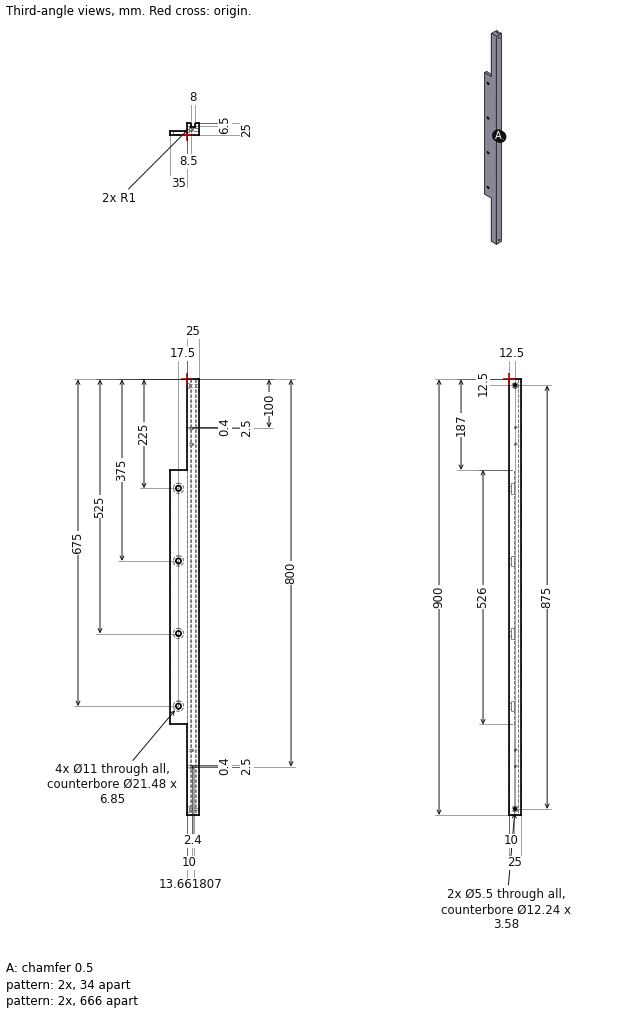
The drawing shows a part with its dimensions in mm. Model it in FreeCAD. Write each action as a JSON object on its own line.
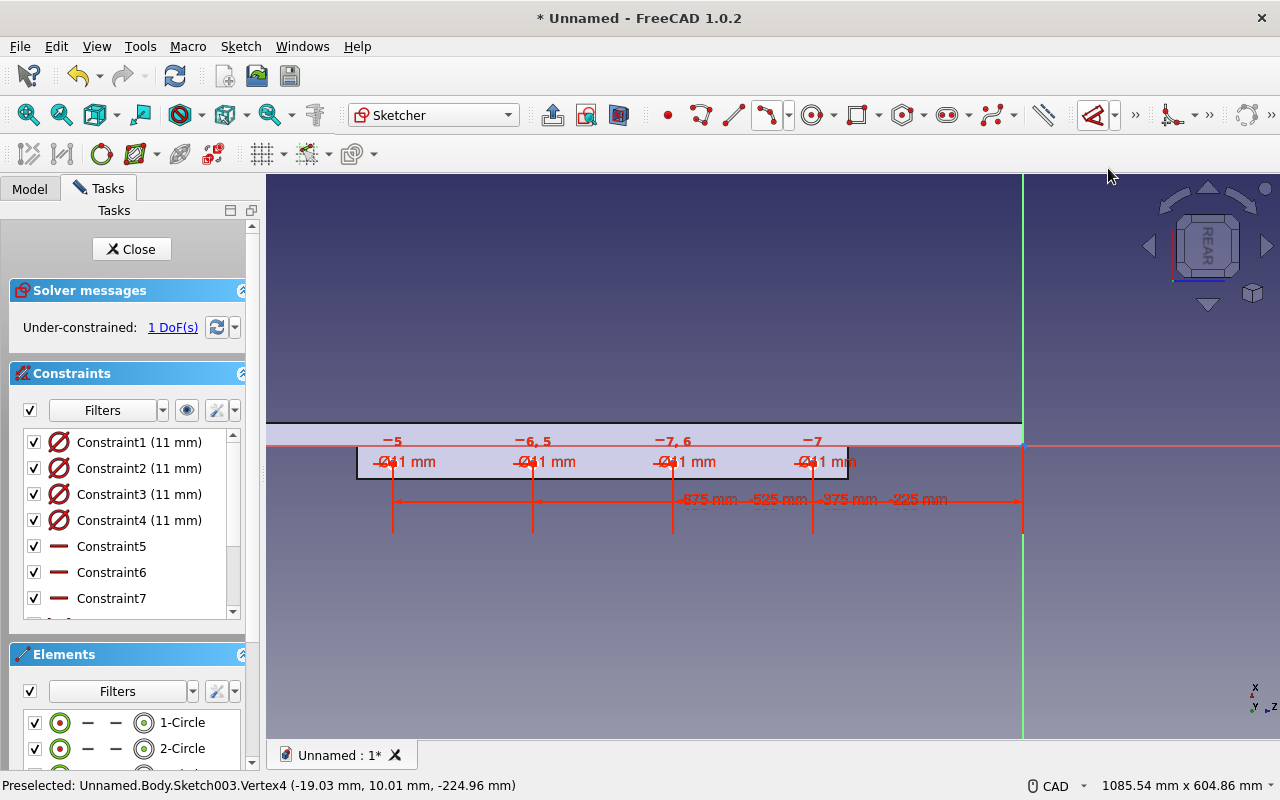
{"action": "scroll", "coordinate": [393, 464], "scroll_direction": "up", "scroll_amount": 5}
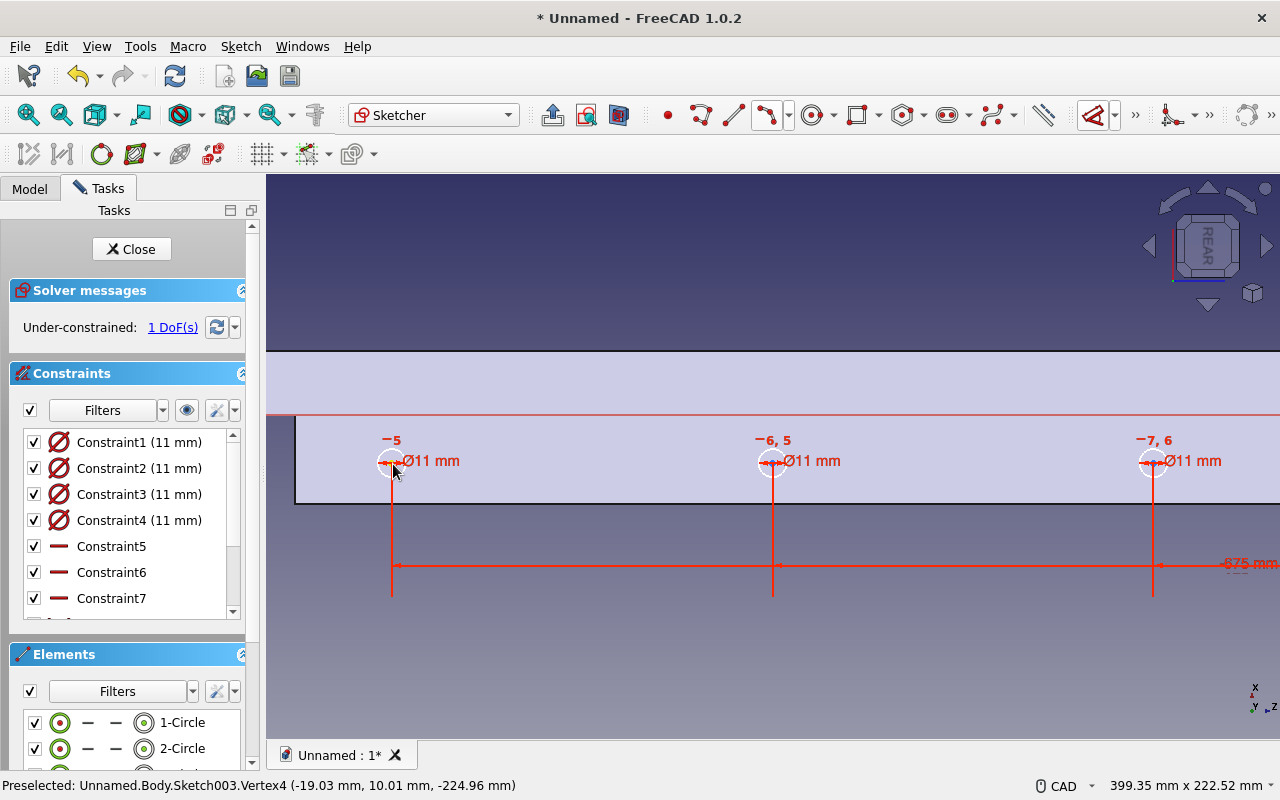
{"action": "left_click", "coordinate": [392, 463]}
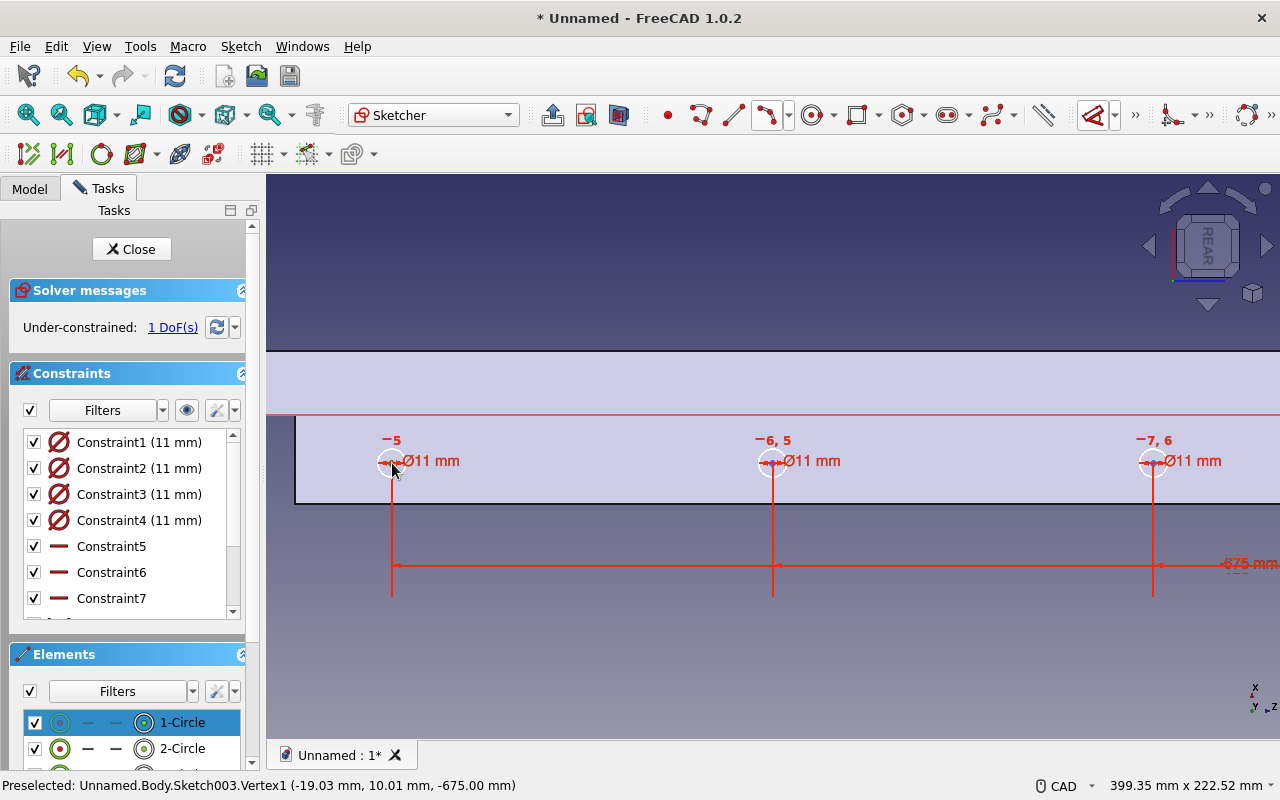
{"action": "left_click", "coordinate": [1114, 116]}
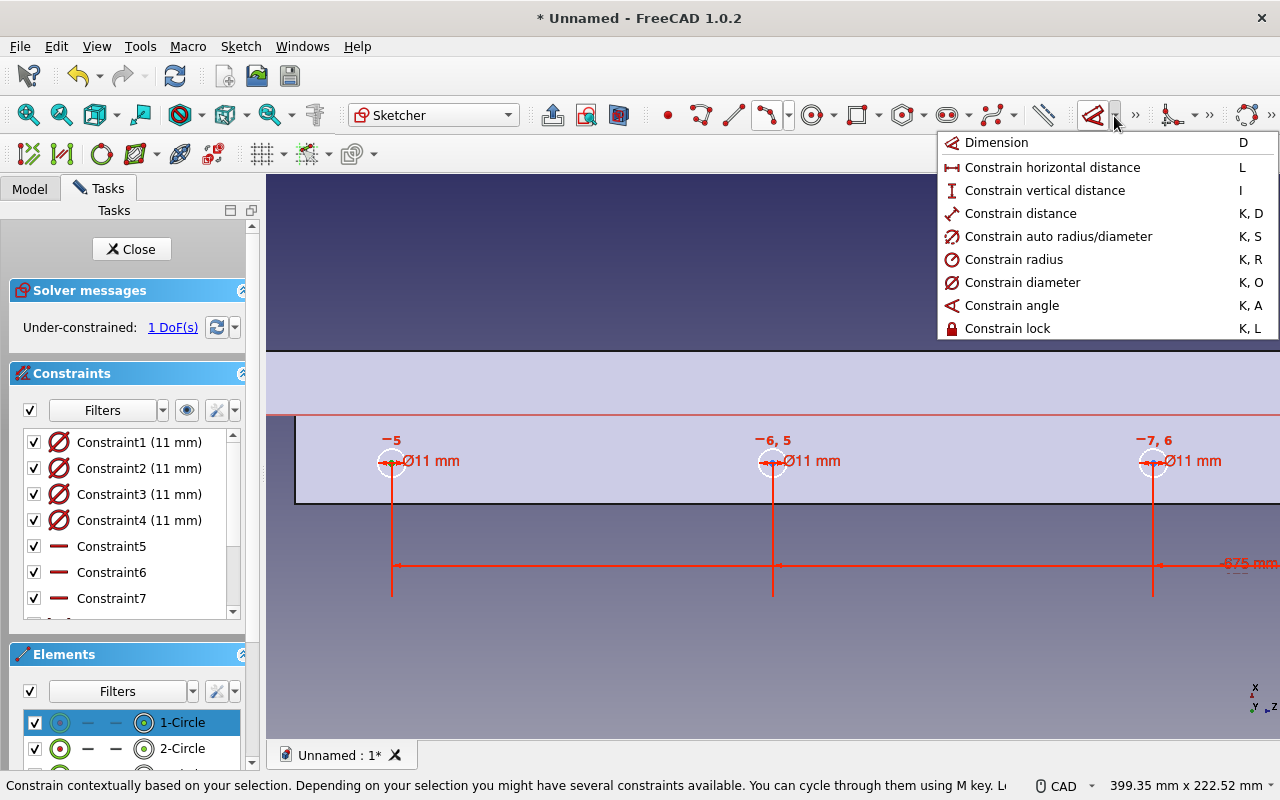
{"action": "left_click", "coordinate": [1108, 190]}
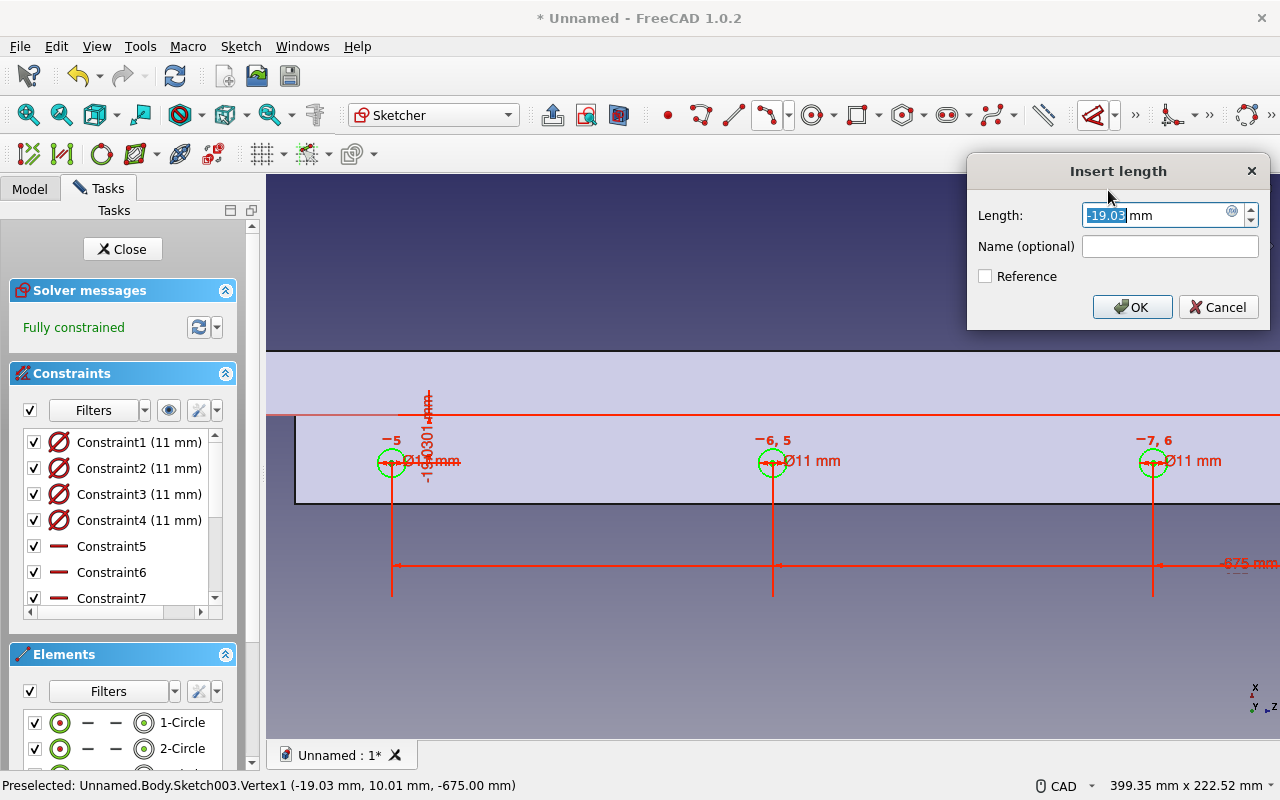
{"action": "type", "text": "-17.5"}
{"action": "key", "text": "Return"}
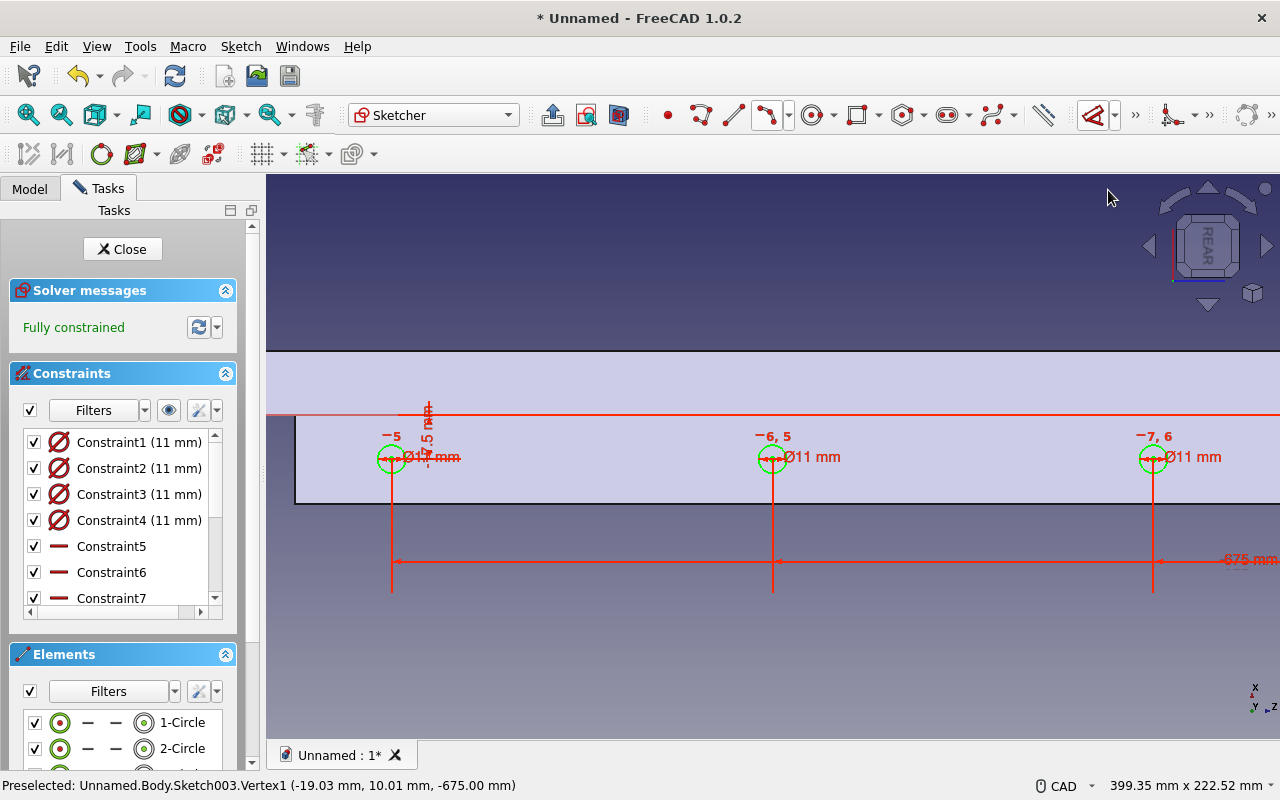
{"action": "left_click", "coordinate": [123, 249]}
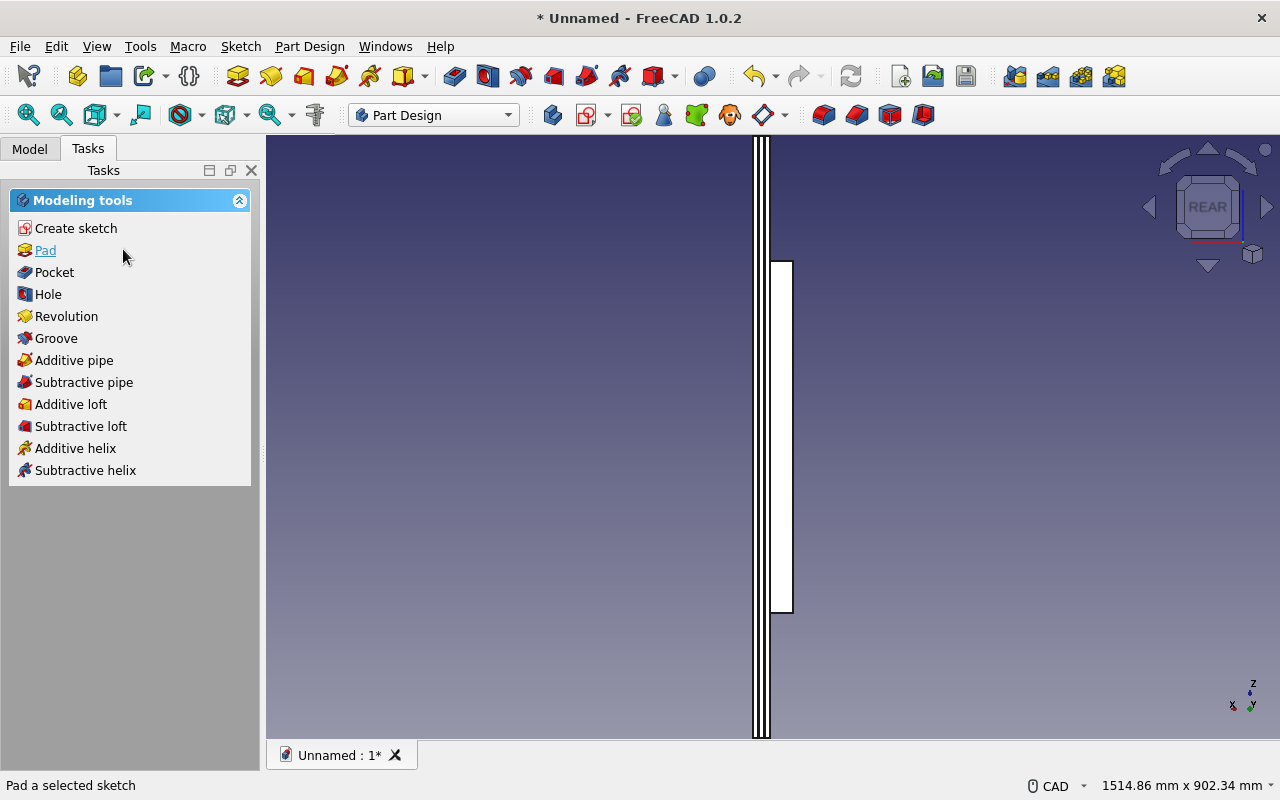
{"action": "left_click", "coordinate": [488, 76]}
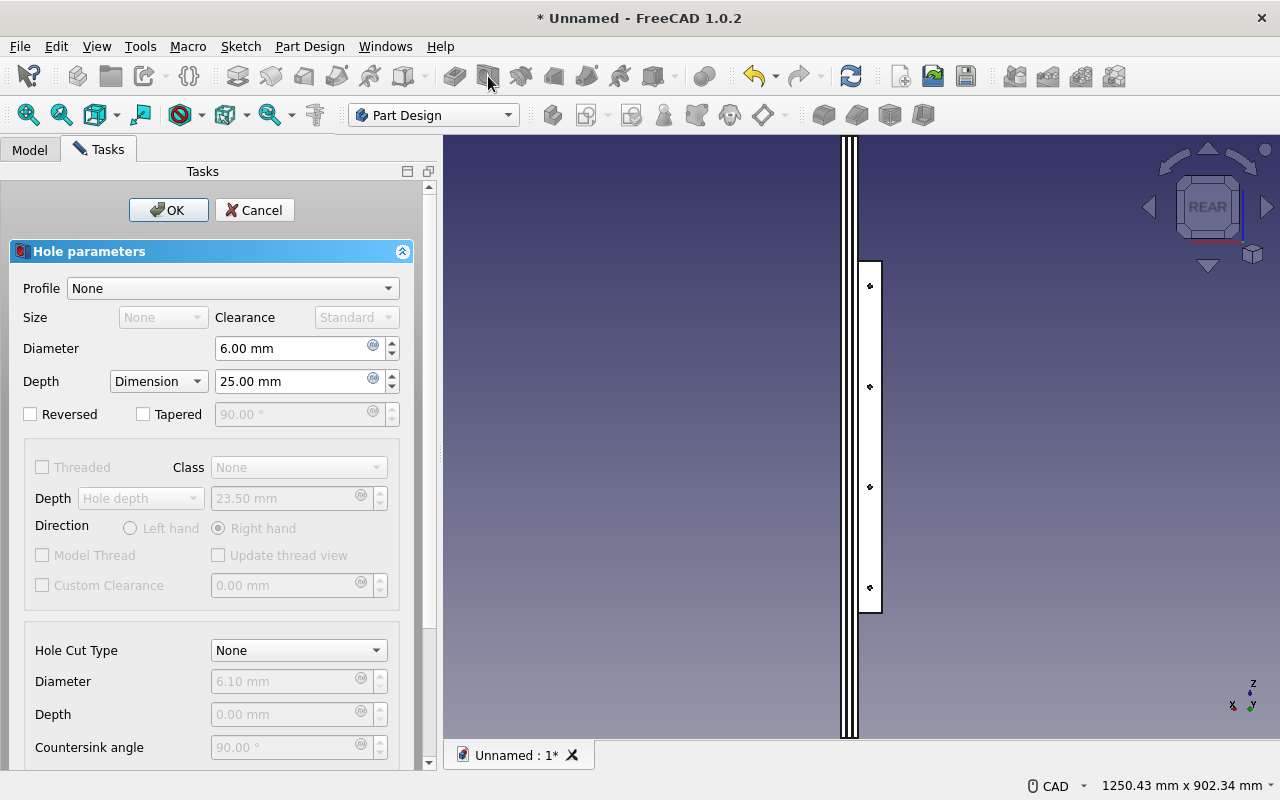
{"action": "triple_click", "coordinate": [300, 348]}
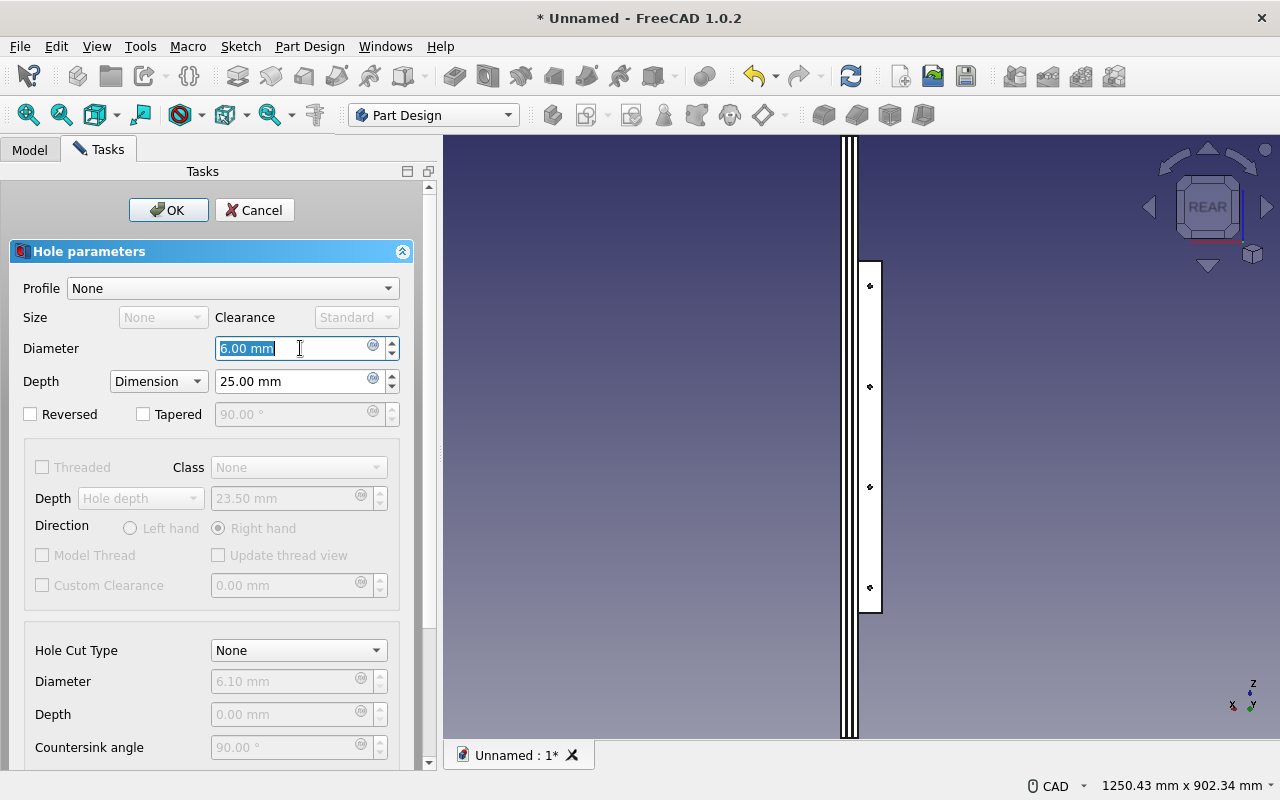
{"action": "type", "text": "11"}
{"action": "key", "text": "Tab"}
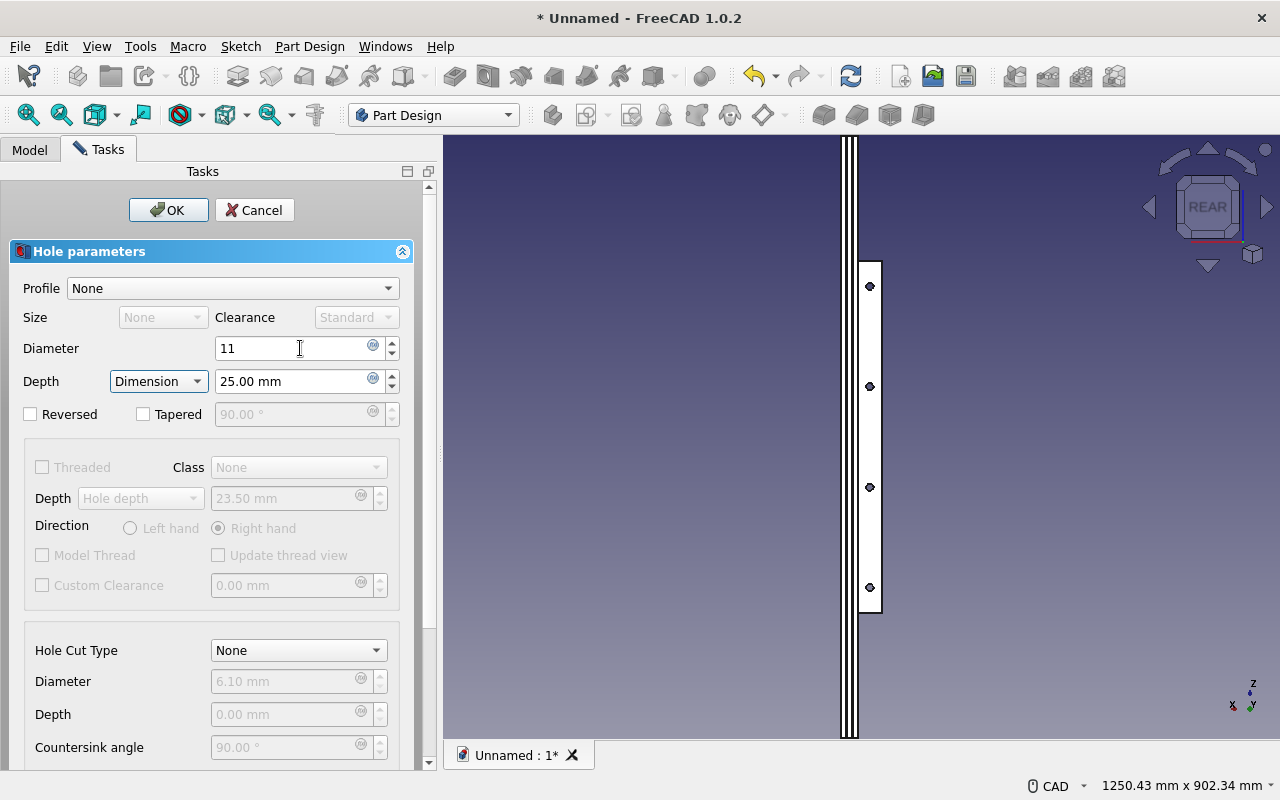
{"action": "left_click", "coordinate": [160, 382]}